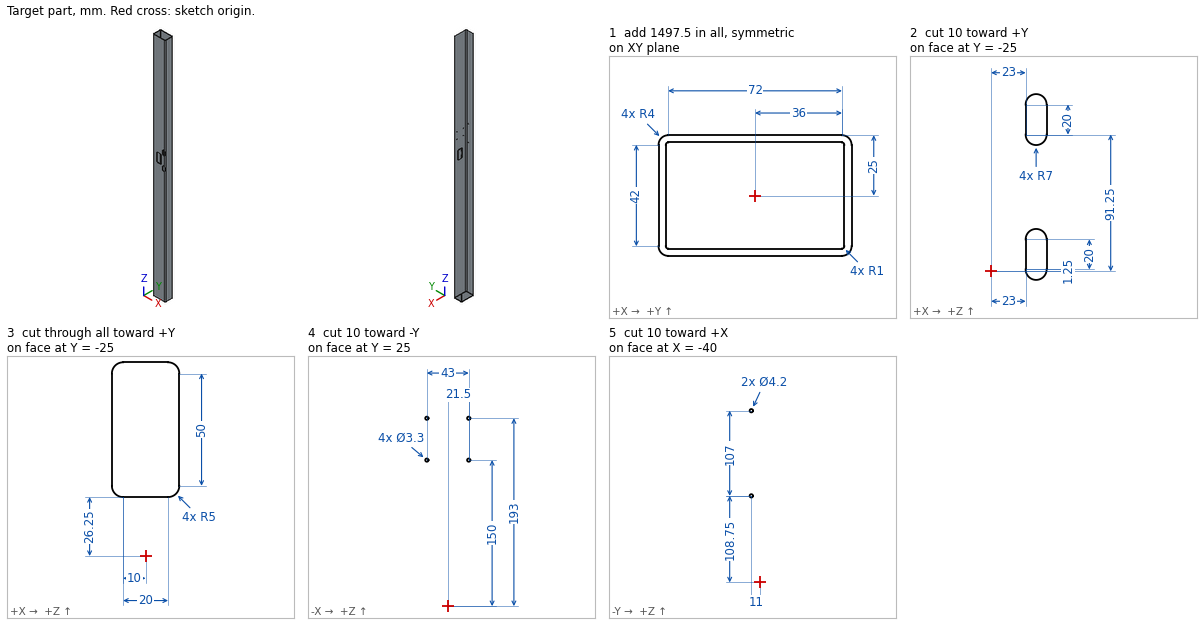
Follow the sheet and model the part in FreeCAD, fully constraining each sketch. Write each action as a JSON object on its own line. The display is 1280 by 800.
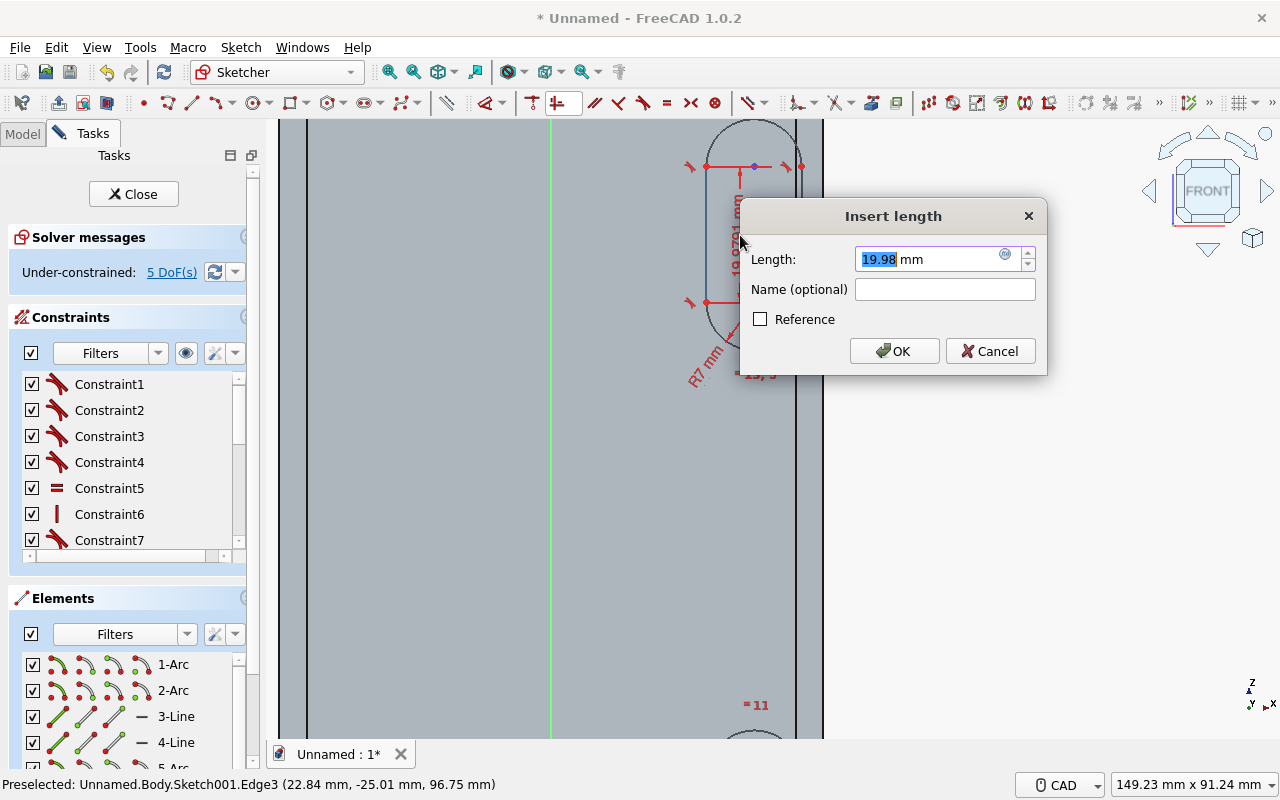
{"action": "type", "text": "20"}
{"action": "key", "text": "Return"}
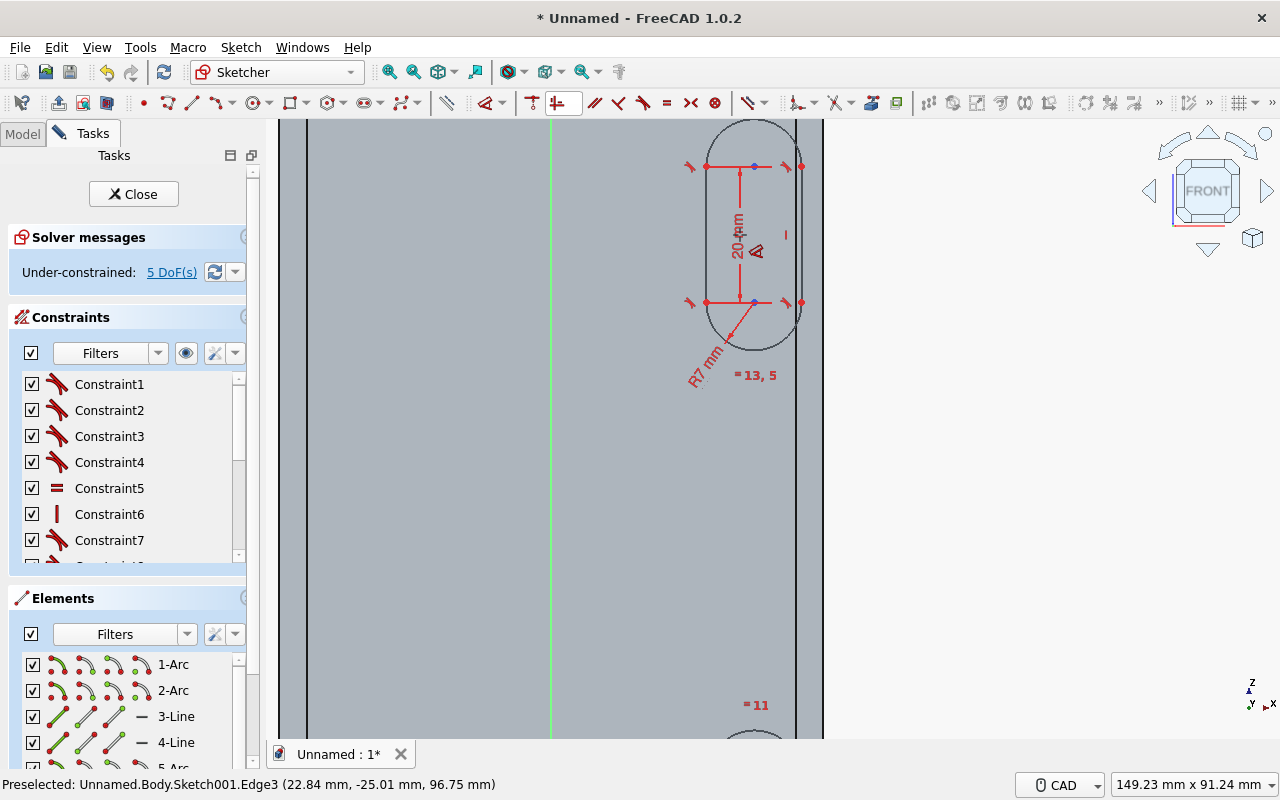
{"action": "scroll", "coordinate": [727, 340], "scroll_direction": "down", "scroll_amount": 4}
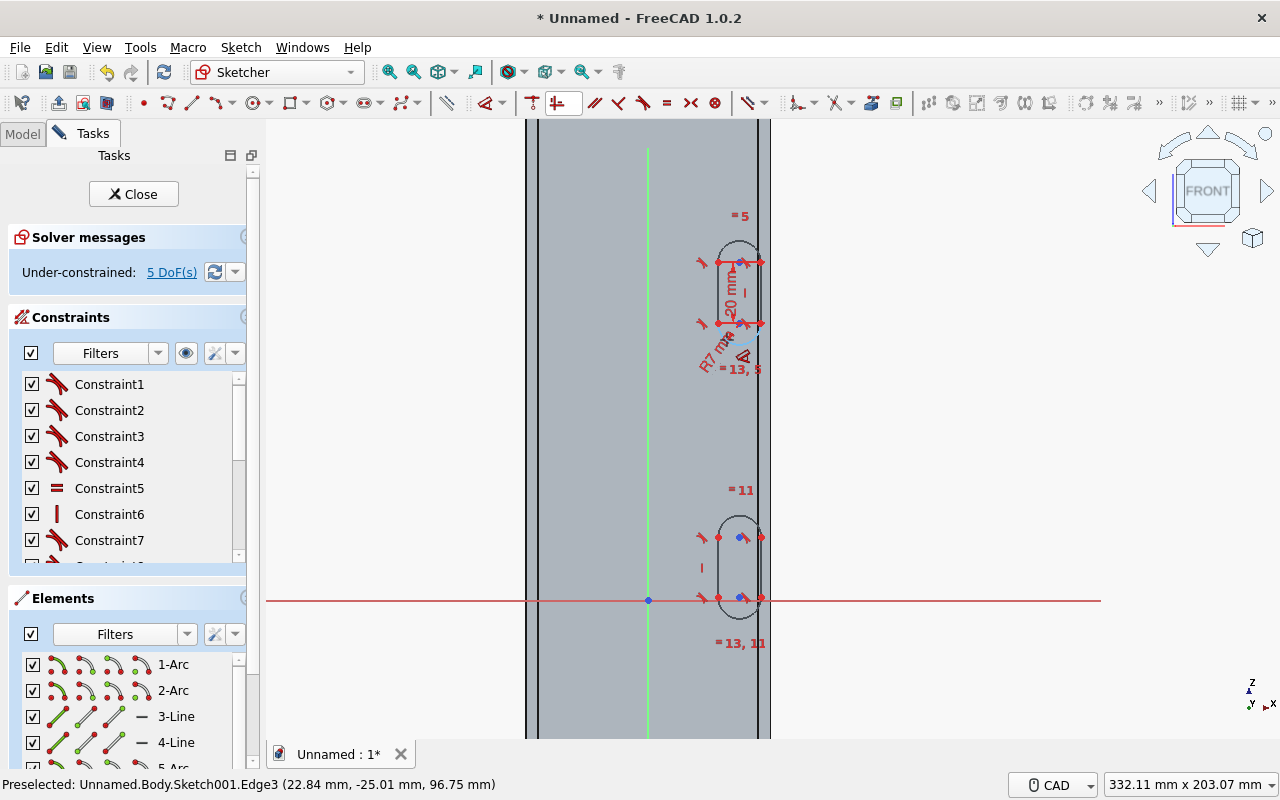
{"action": "left_click", "coordinate": [718, 579]}
{"action": "left_click", "coordinate": [684, 567]}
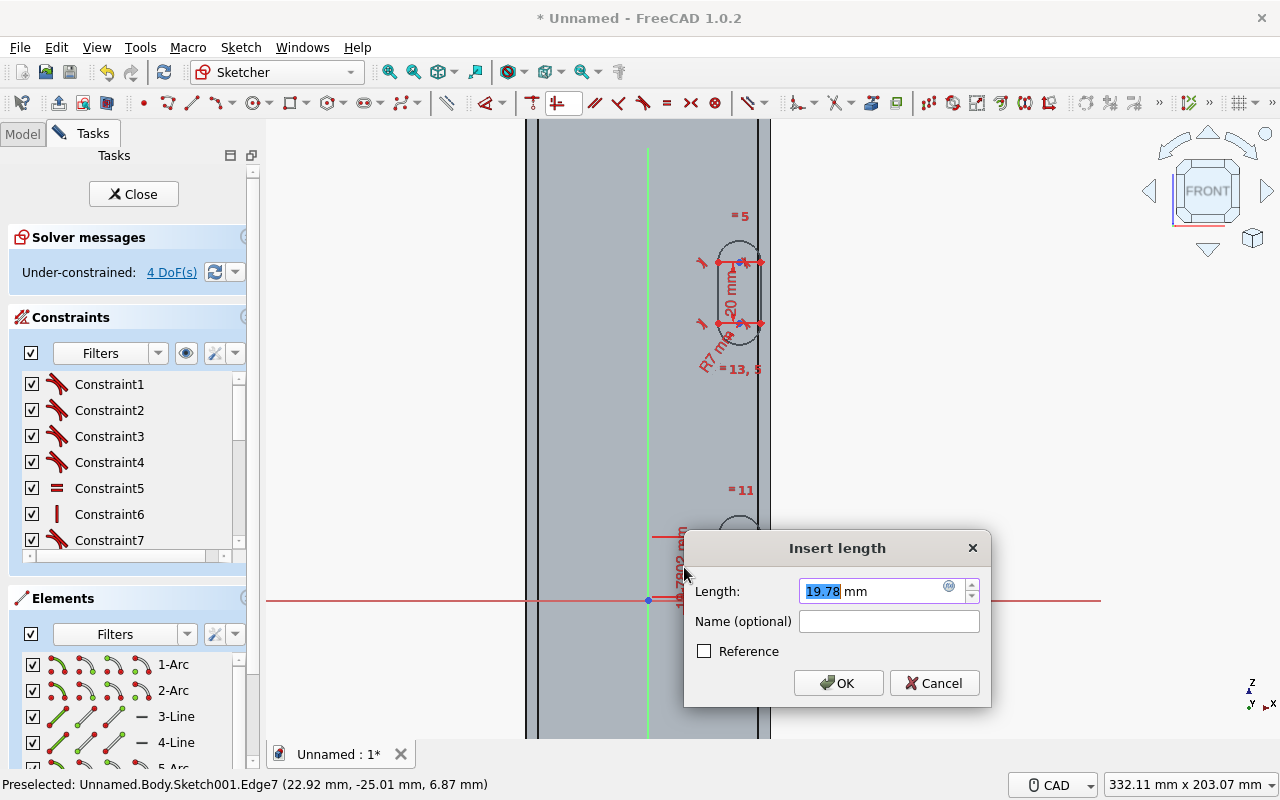
{"action": "type", "text": "20"}
{"action": "key", "text": "Return"}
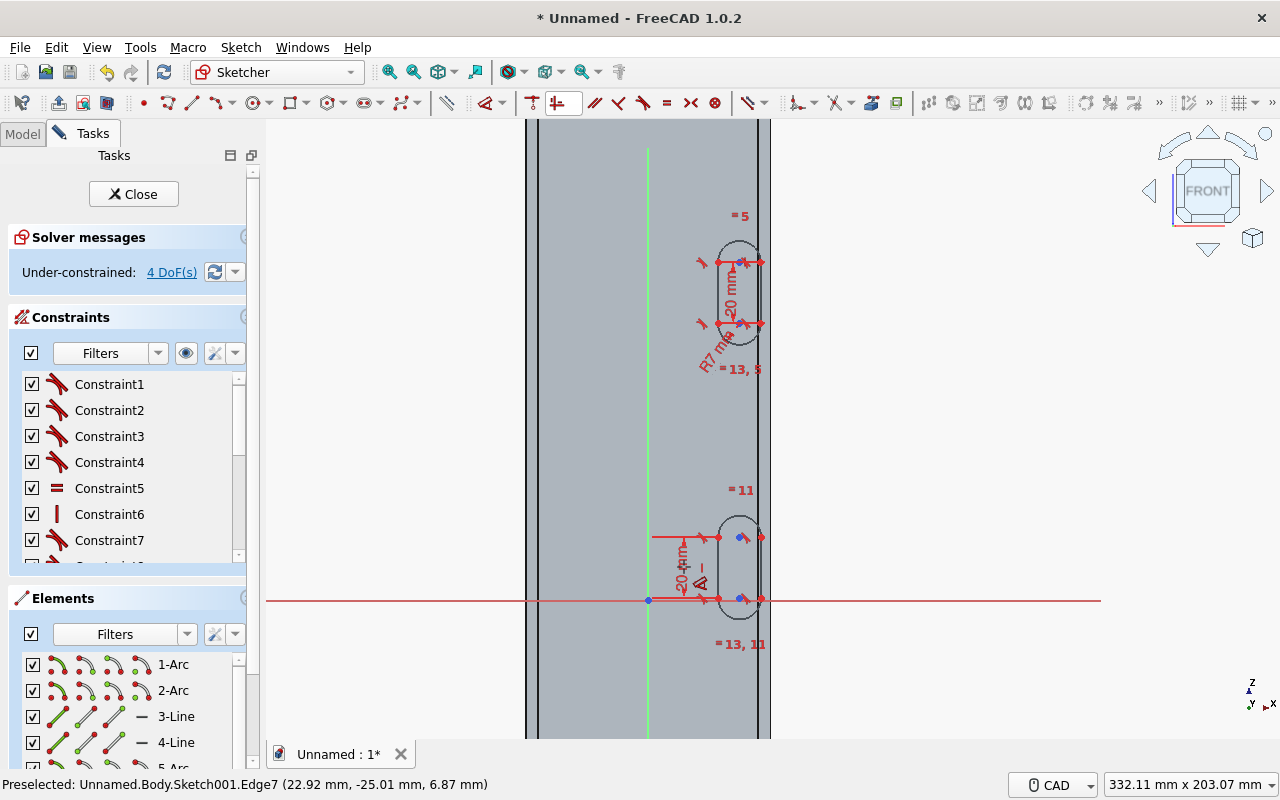
{"action": "left_click", "coordinate": [718, 323]}
{"action": "left_click", "coordinate": [683, 635]}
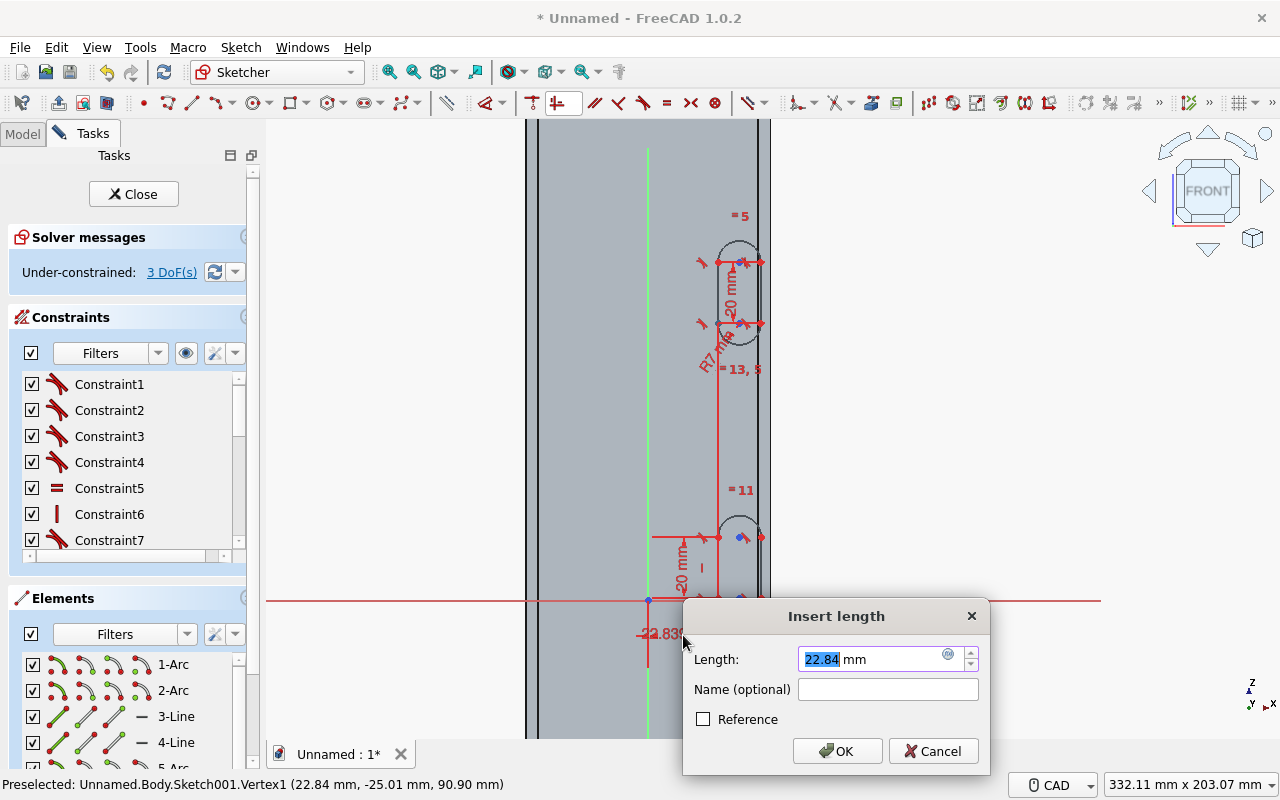
{"action": "type", "text": "23"}
{"action": "key", "text": "Return"}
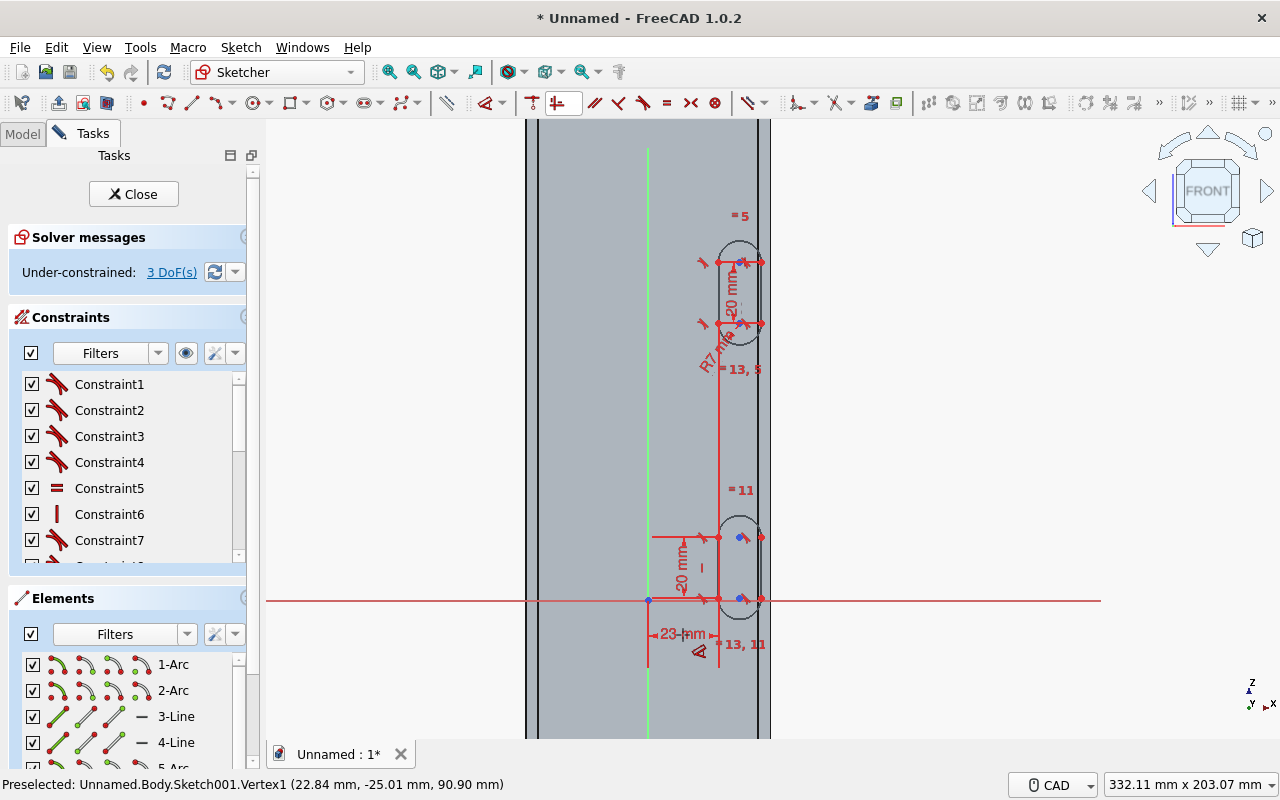
{"action": "left_click", "coordinate": [718, 598]}
{"action": "left_click", "coordinate": [683, 659]}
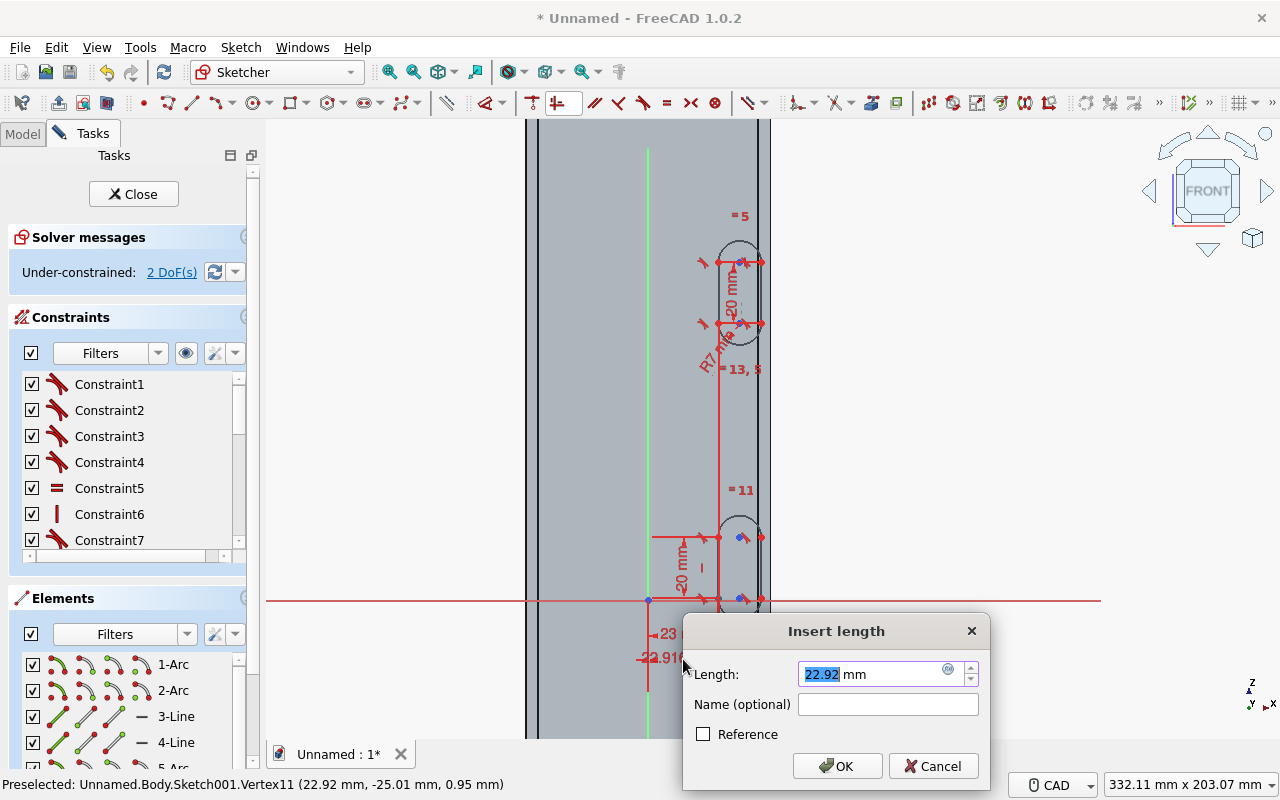
{"action": "type", "text": "23"}
{"action": "key", "text": "Return"}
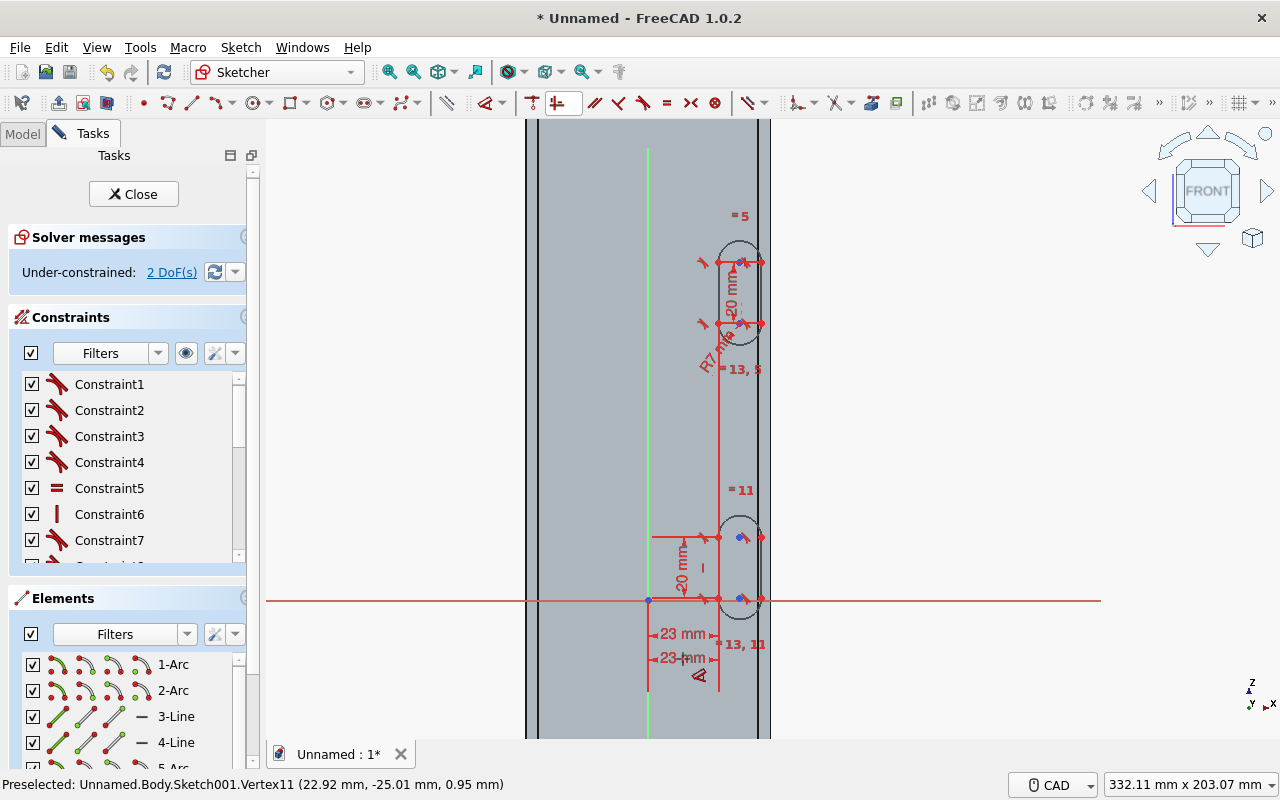
{"action": "scroll", "coordinate": [719, 598], "scroll_direction": "up", "scroll_amount": 12}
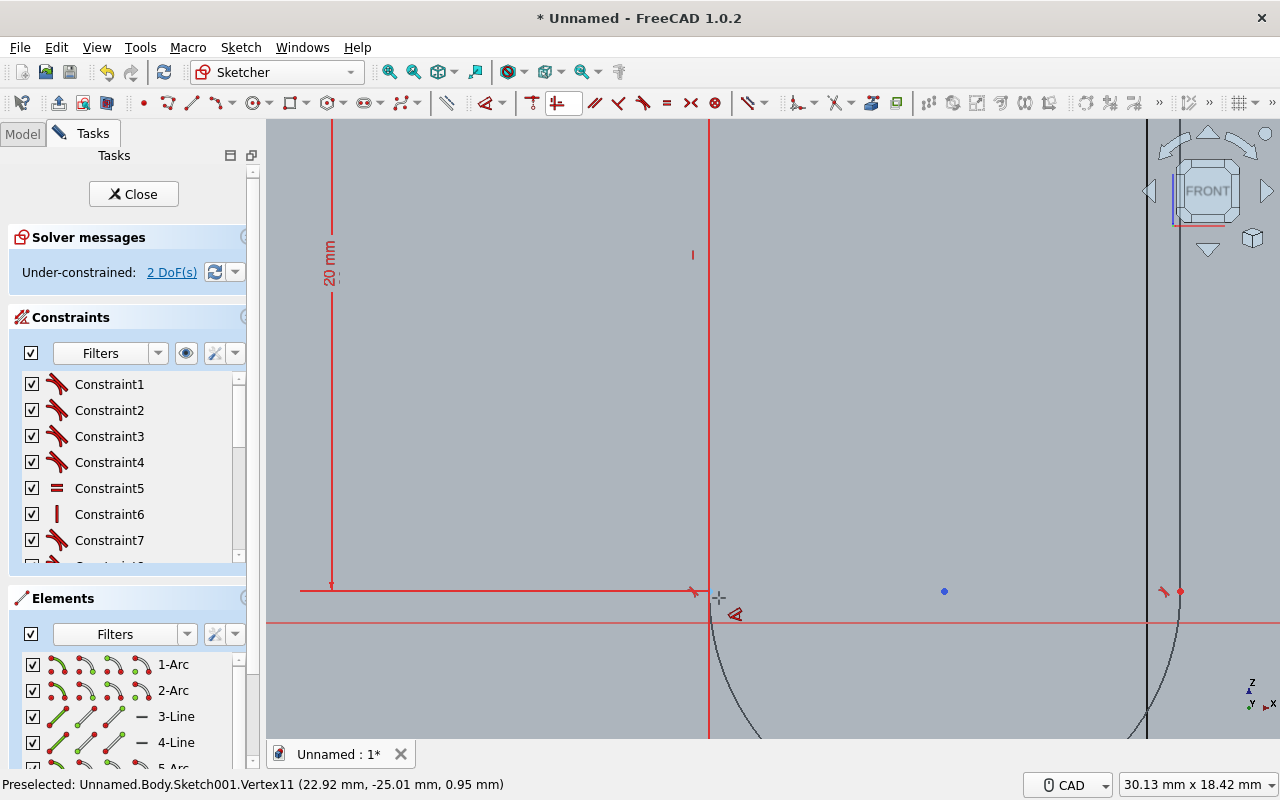
{"action": "left_click", "coordinate": [709, 591]}
{"action": "left_click", "coordinate": [743, 607]}